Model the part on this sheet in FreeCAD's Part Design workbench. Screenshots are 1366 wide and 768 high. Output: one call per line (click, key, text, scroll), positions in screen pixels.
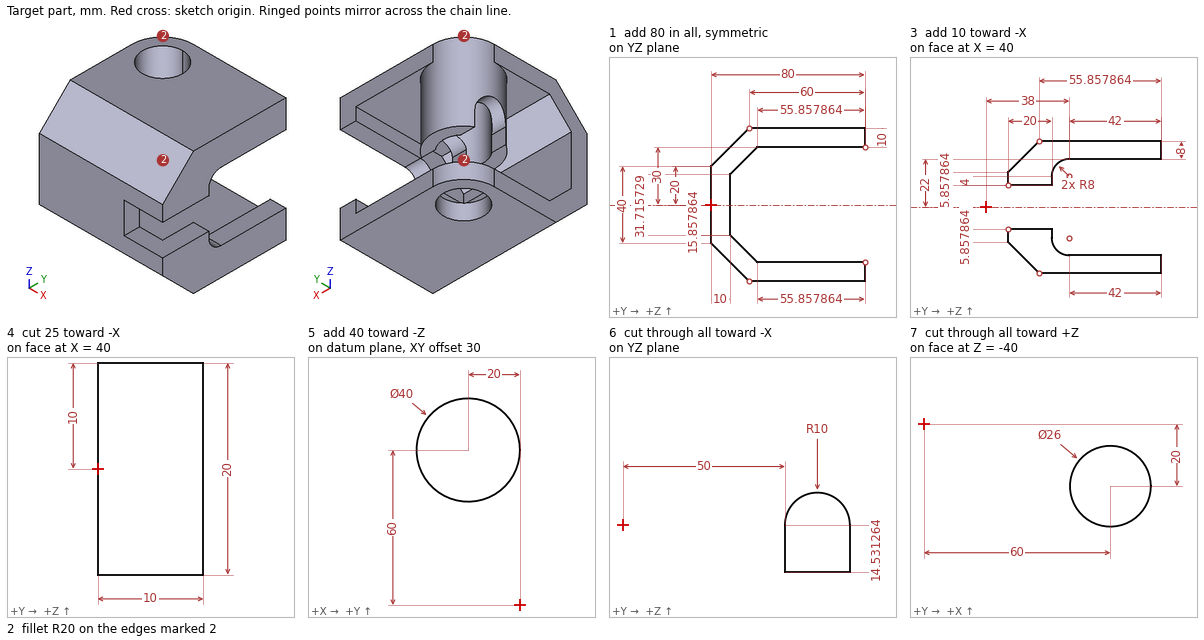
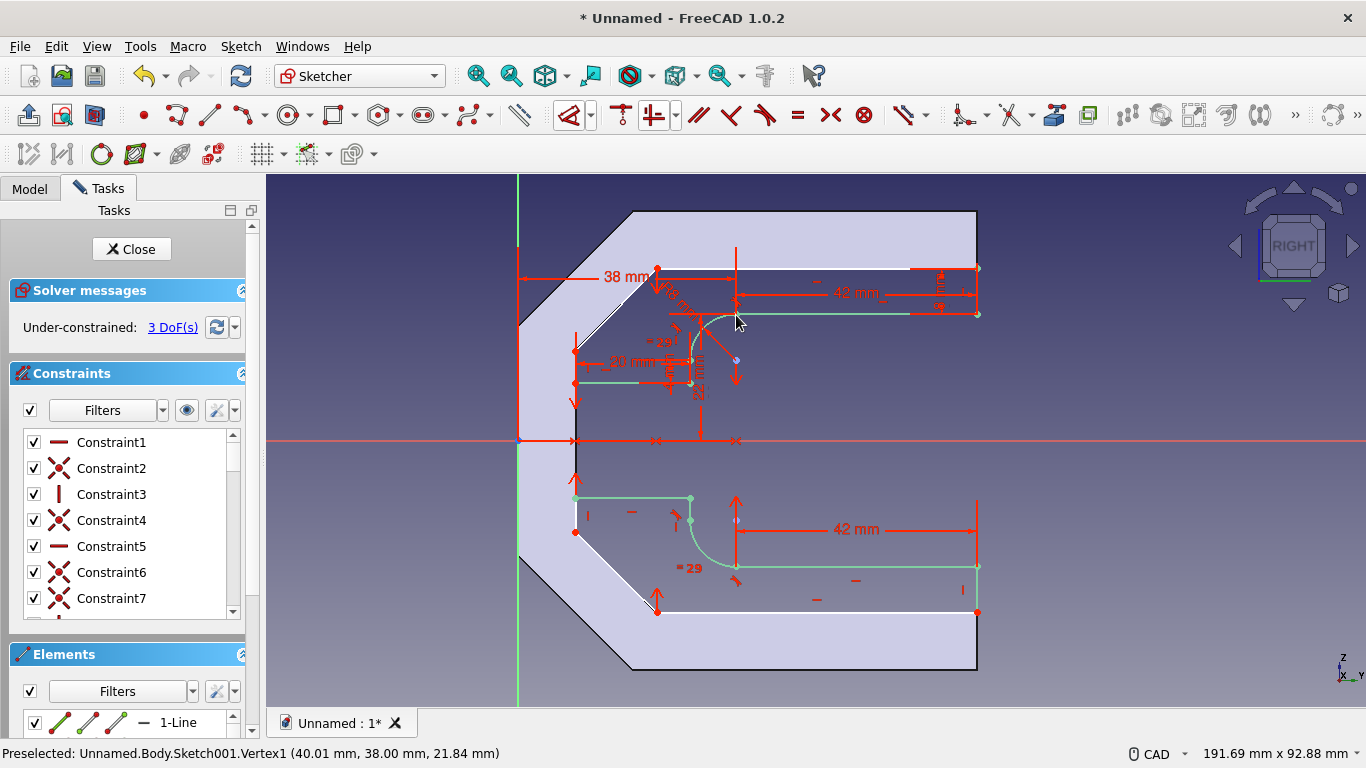
scroll(576, 361, up, 2)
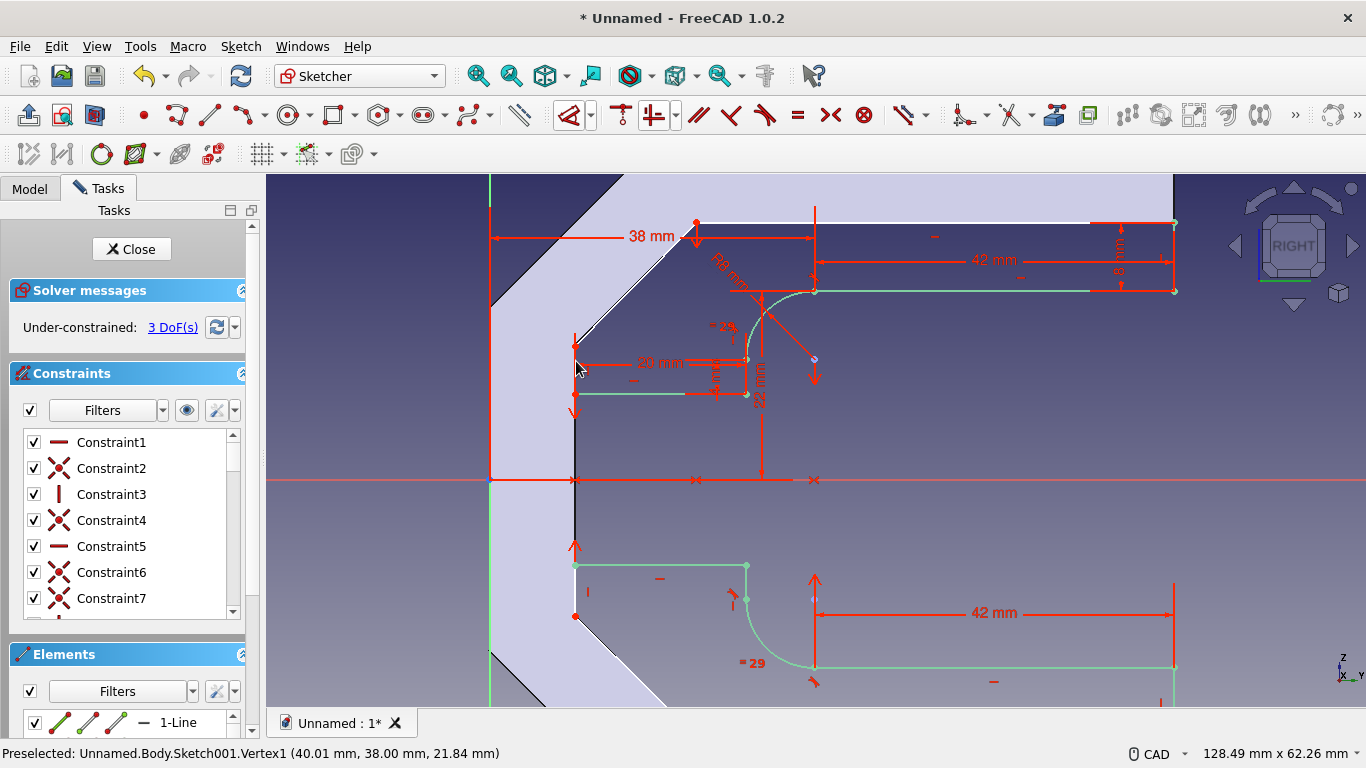
click(575, 361)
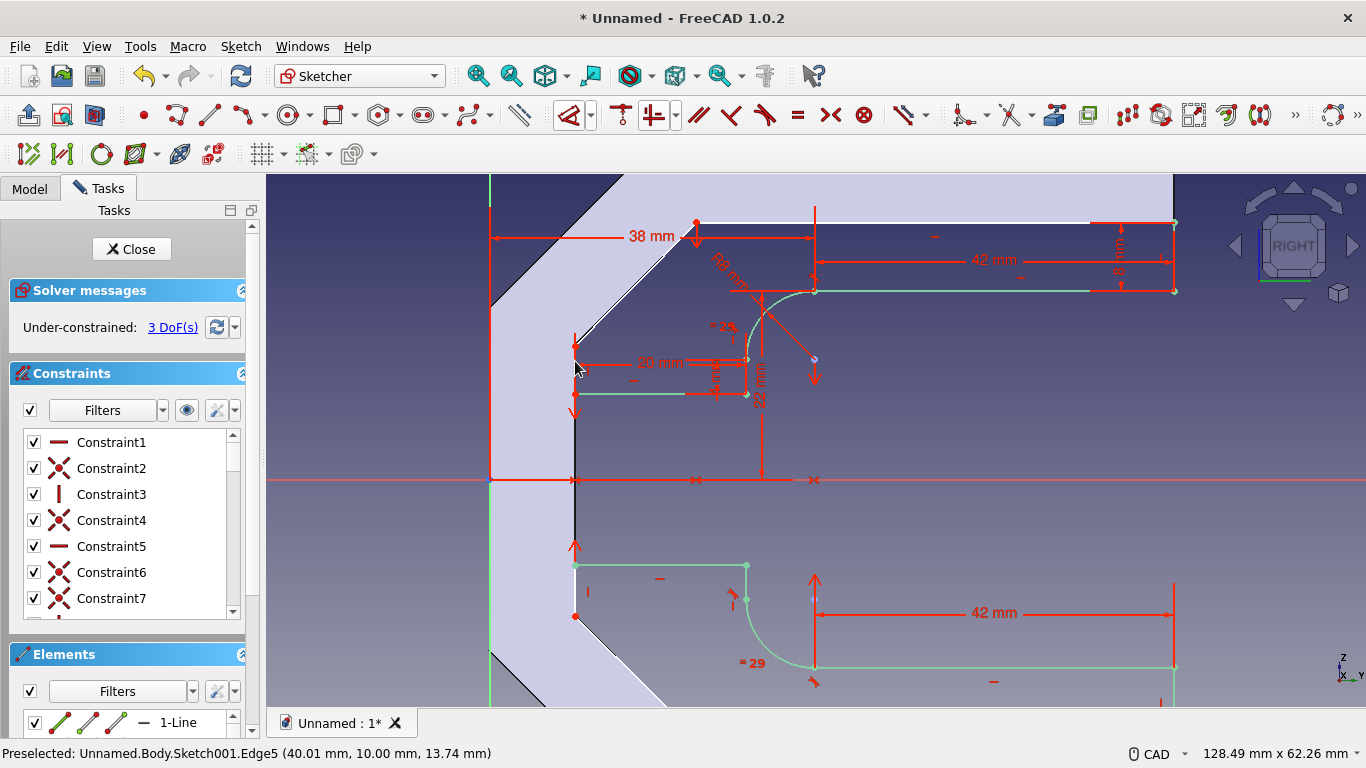
click(590, 116)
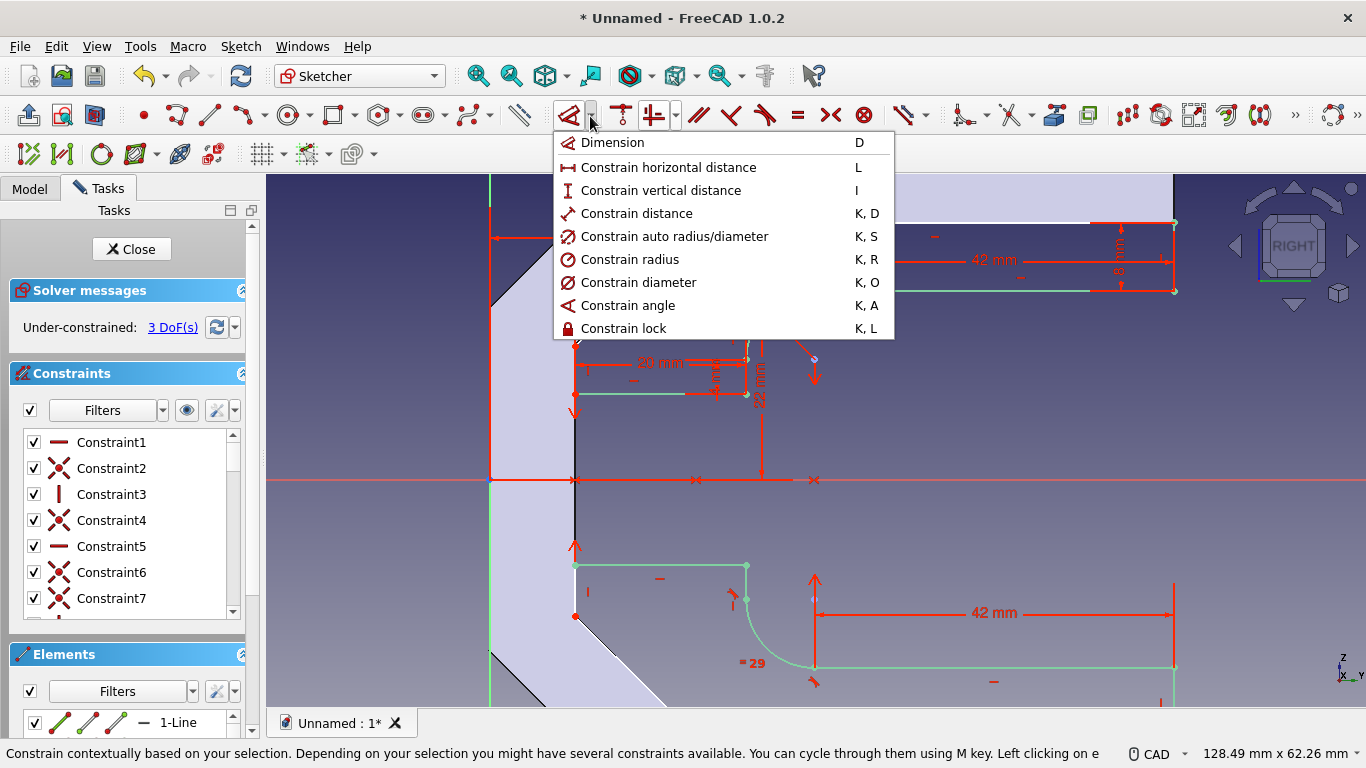
click(724, 190)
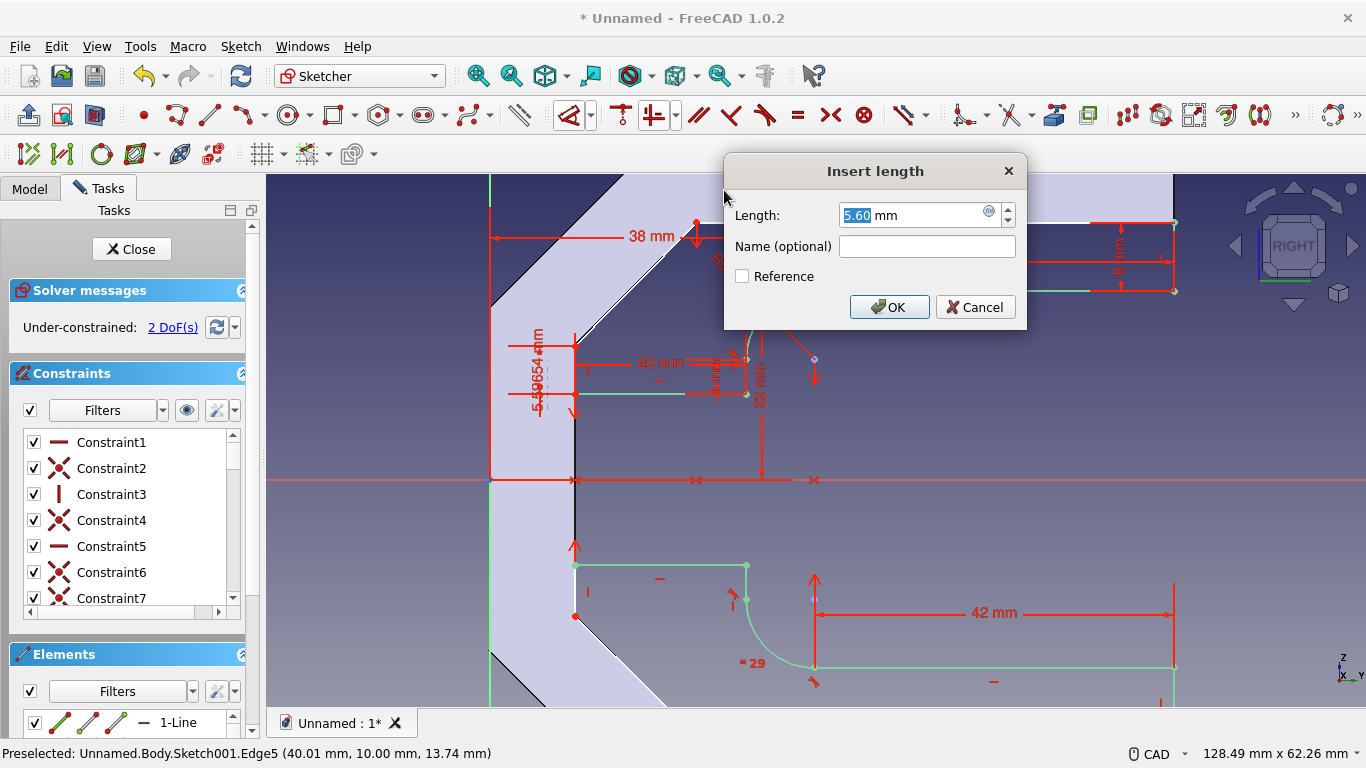
text(5.857864)
key(Return)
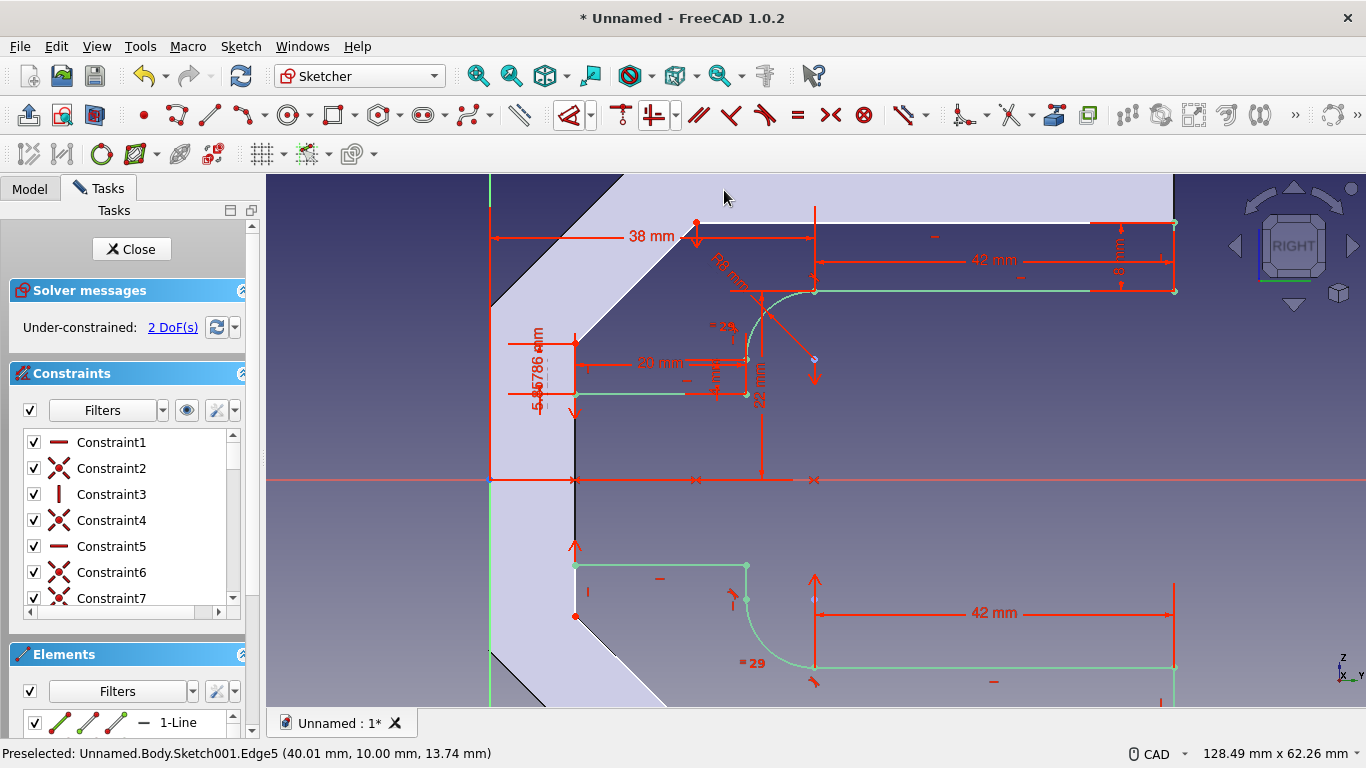
click(575, 581)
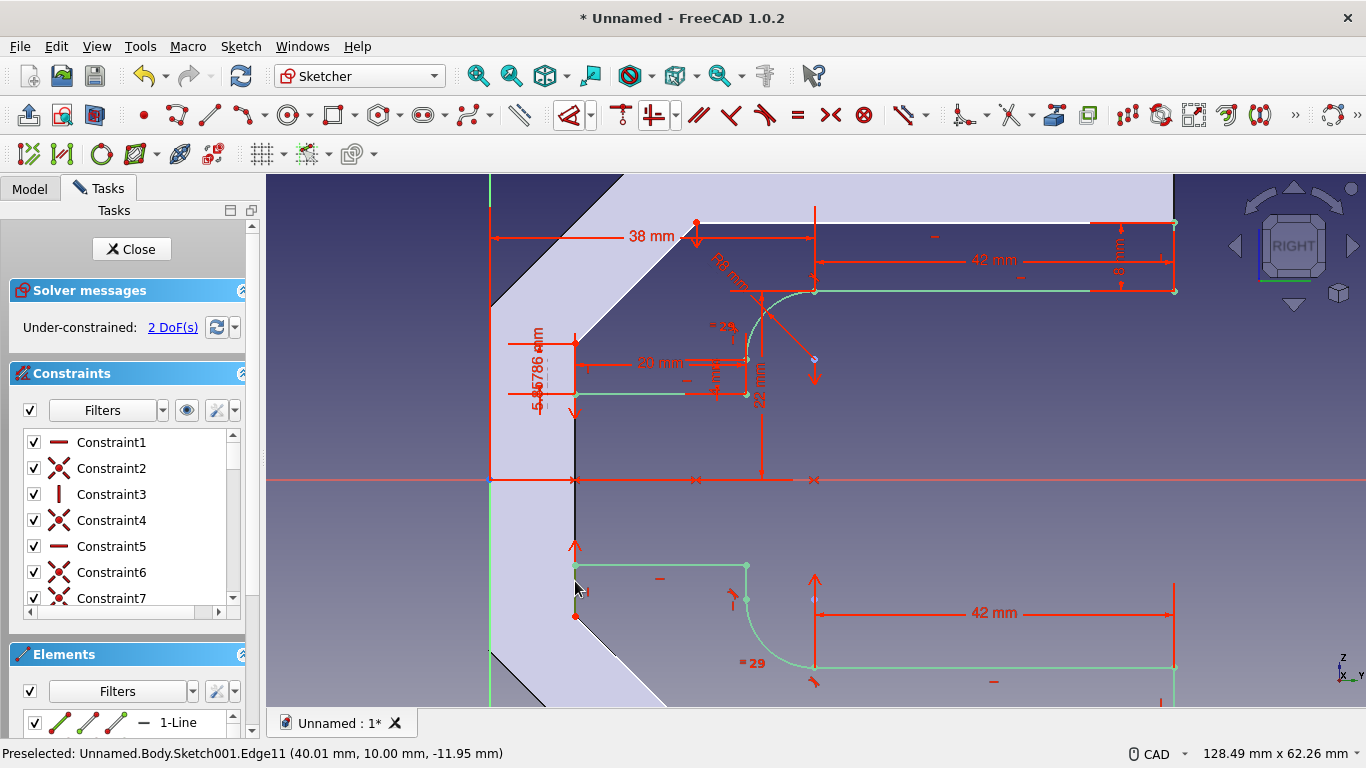
click(590, 116)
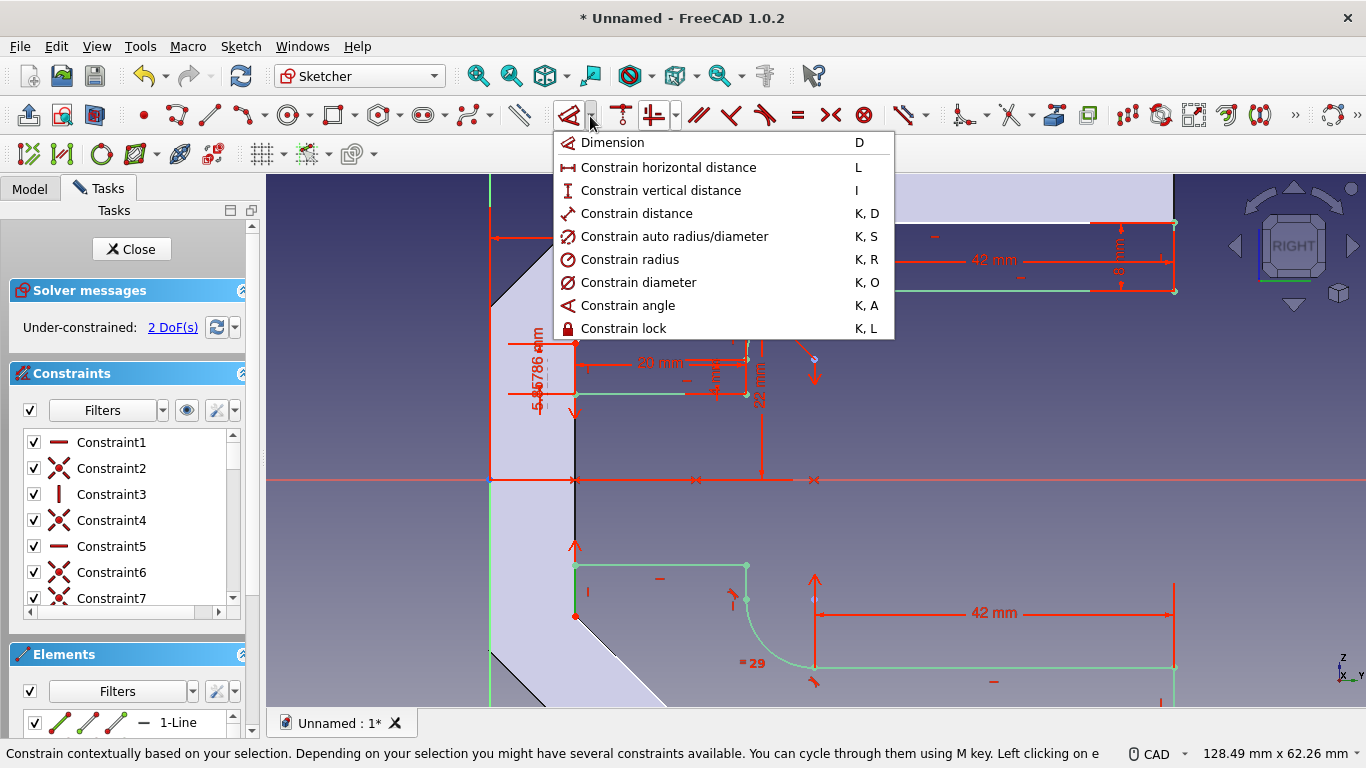
click(724, 190)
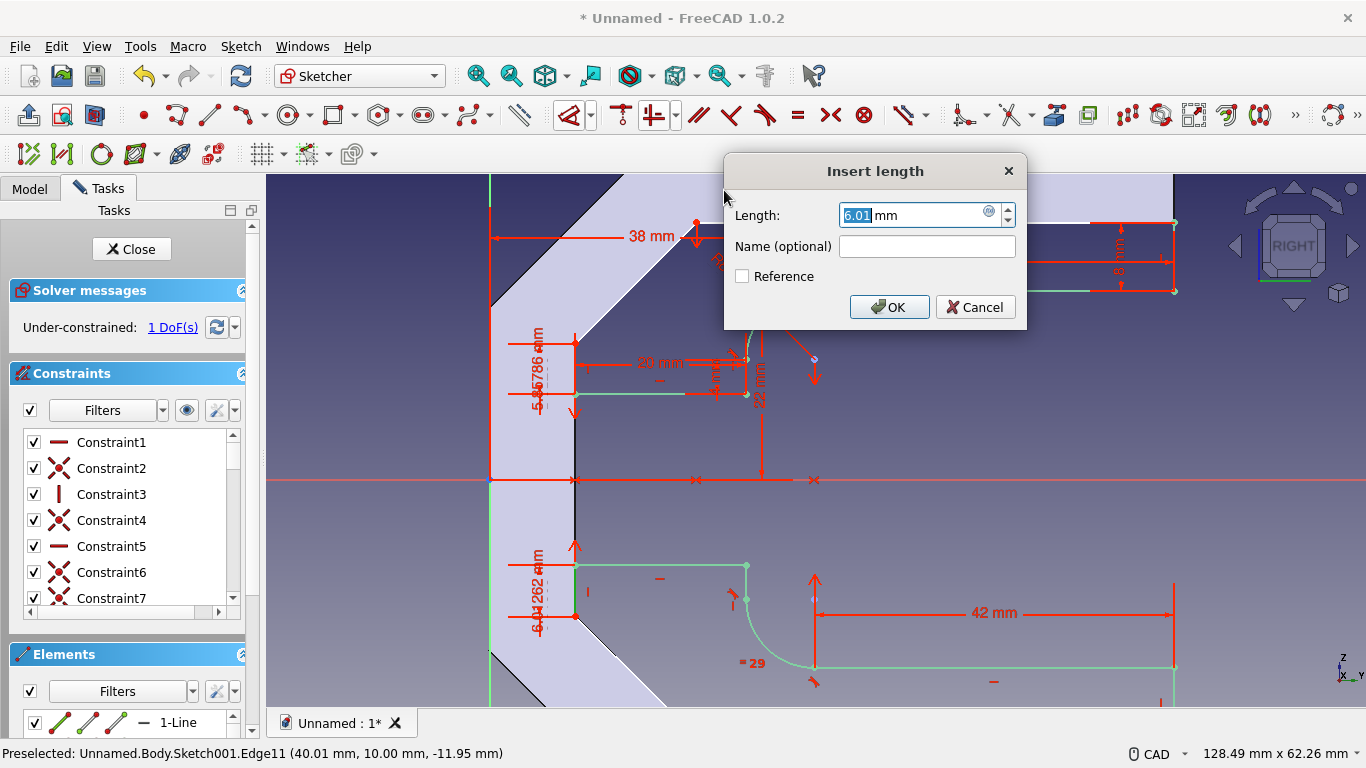
text(5.857864)
key(Return)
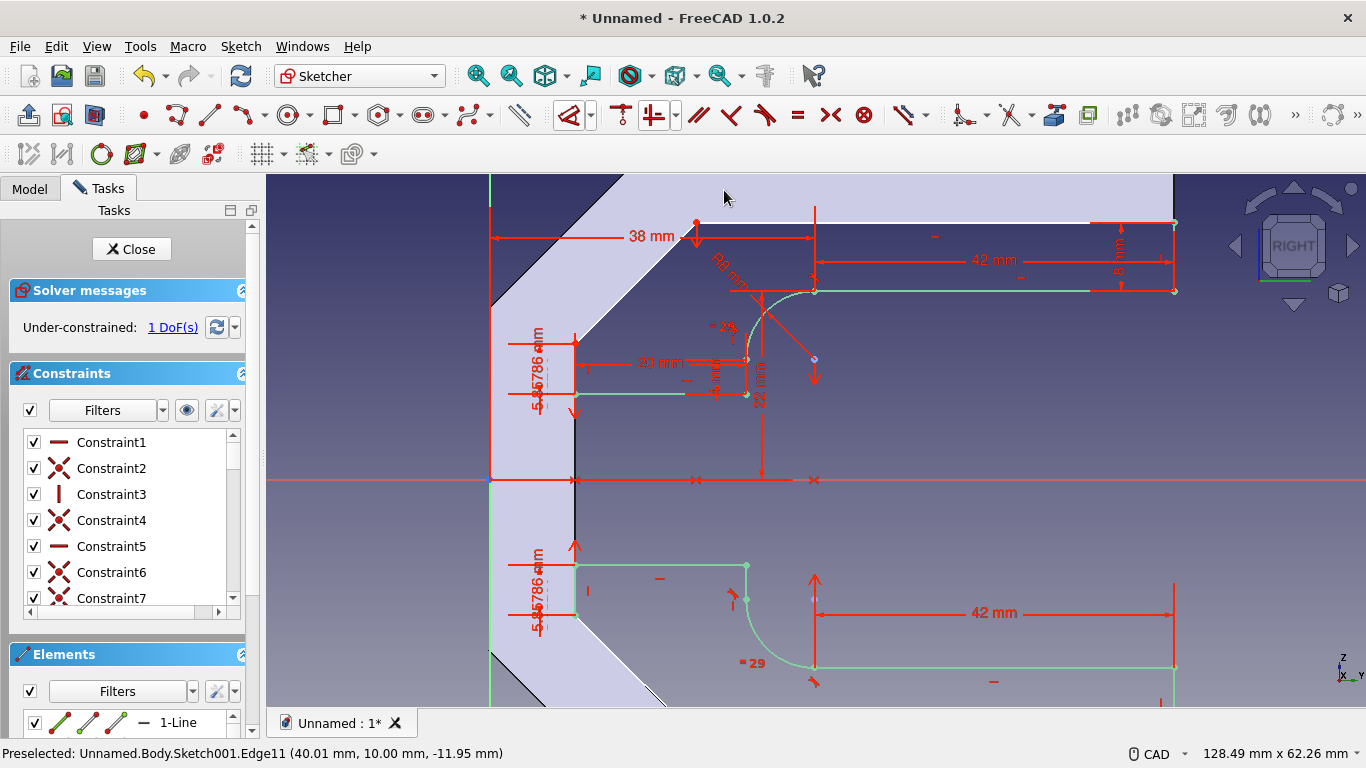
click(1031, 223)